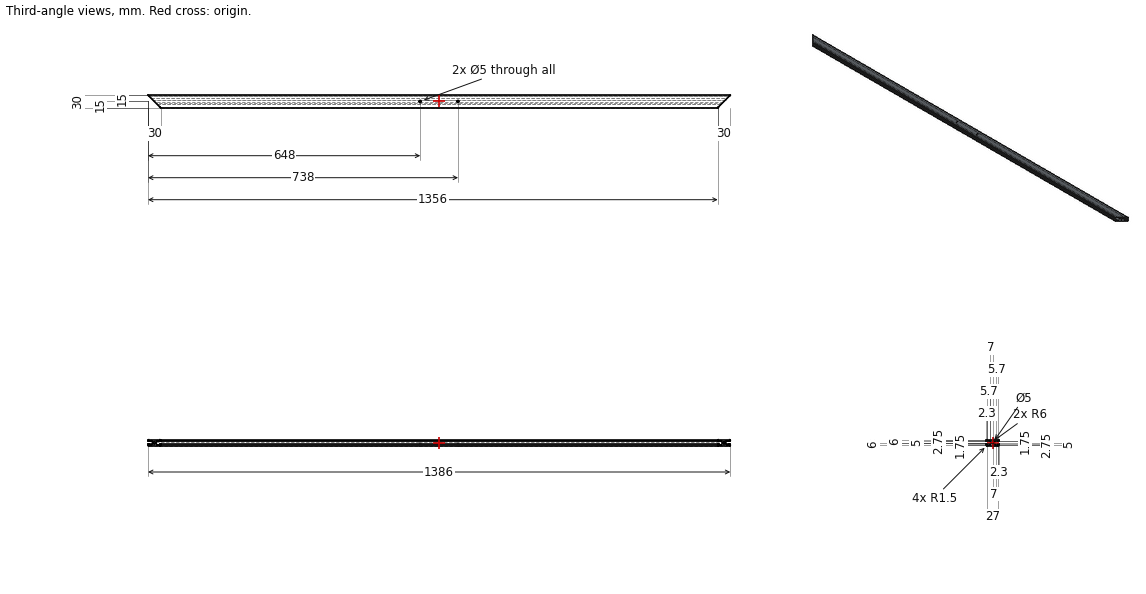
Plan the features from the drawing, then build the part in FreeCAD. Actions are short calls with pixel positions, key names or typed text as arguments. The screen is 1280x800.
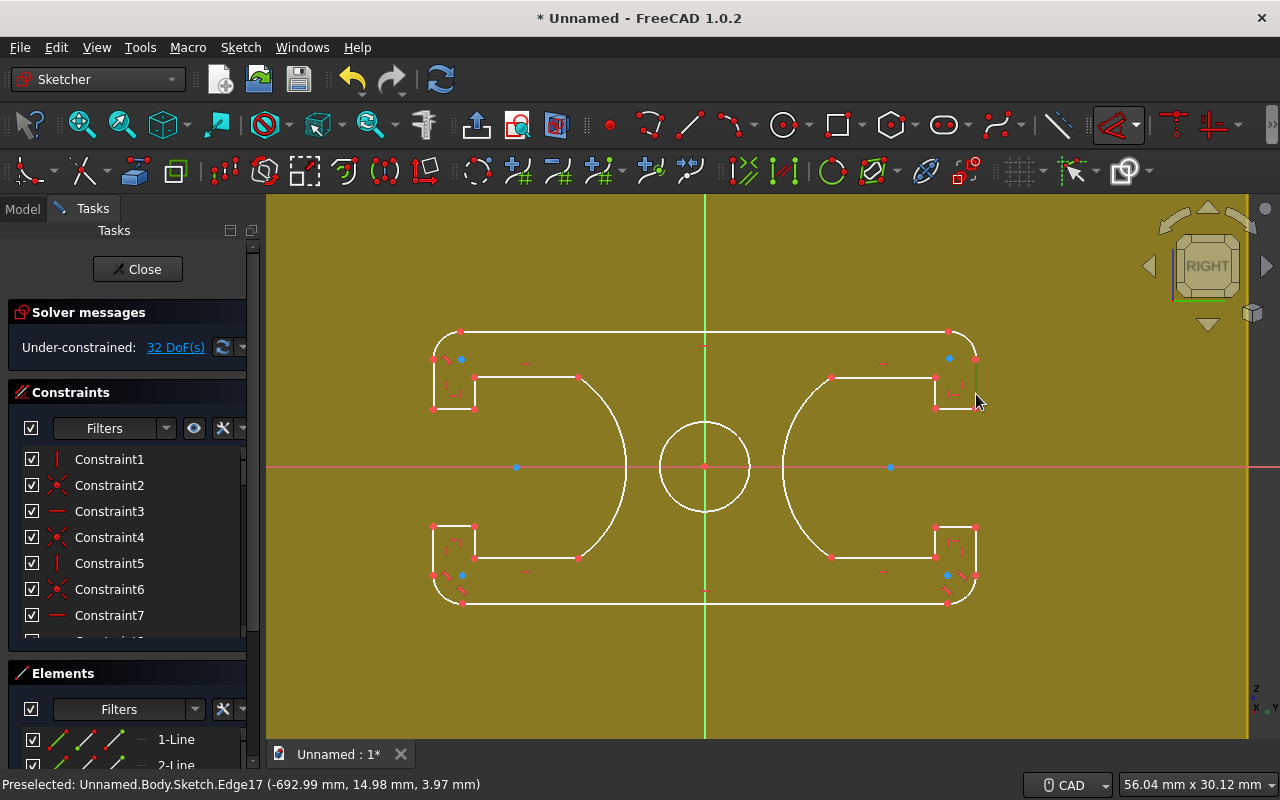
click(973, 347)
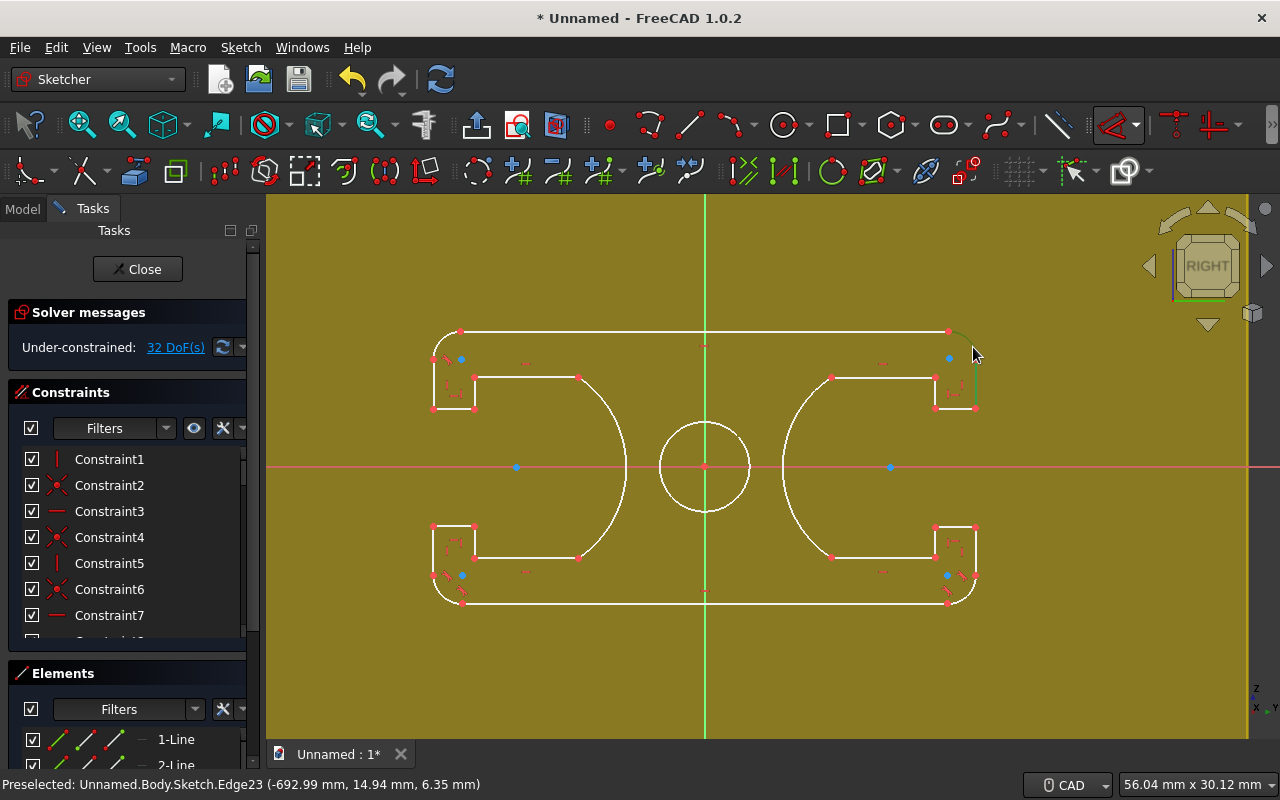
key(t)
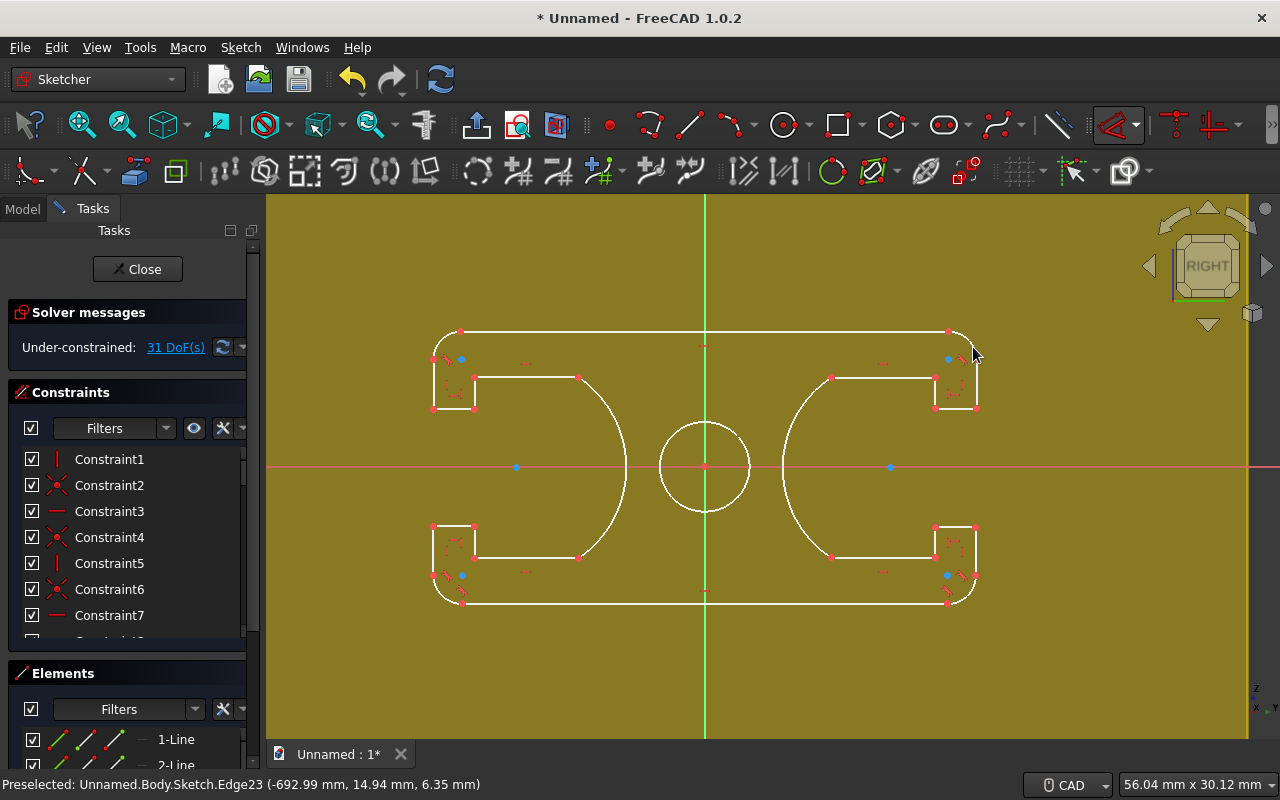
click(803, 332)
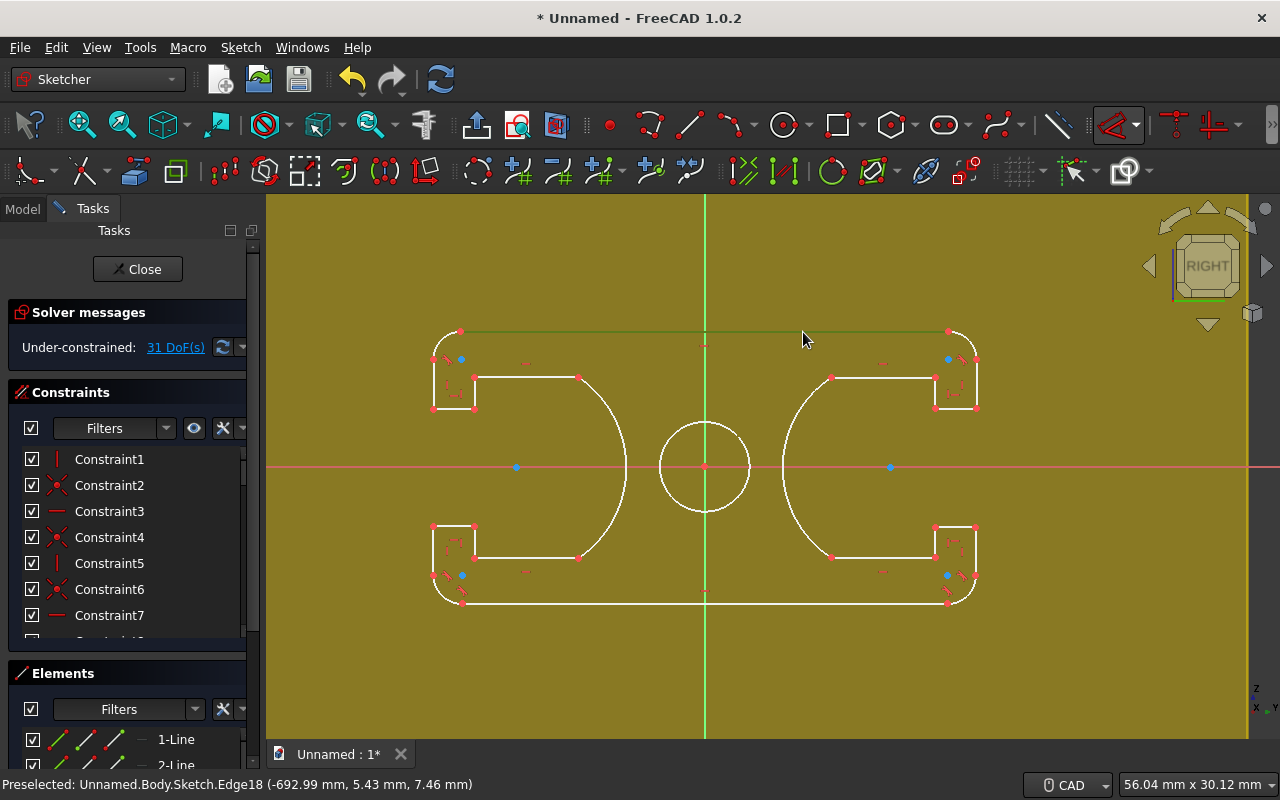
click(974, 347)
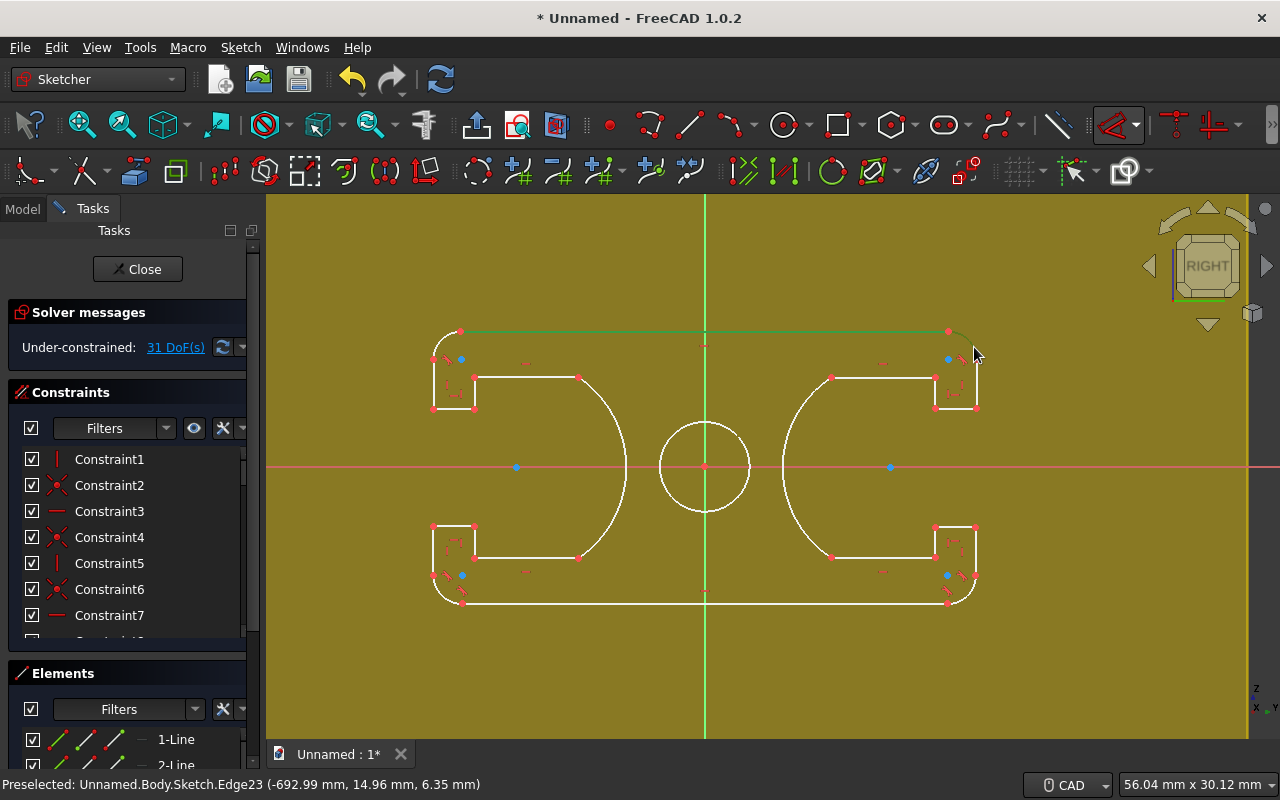
key(t)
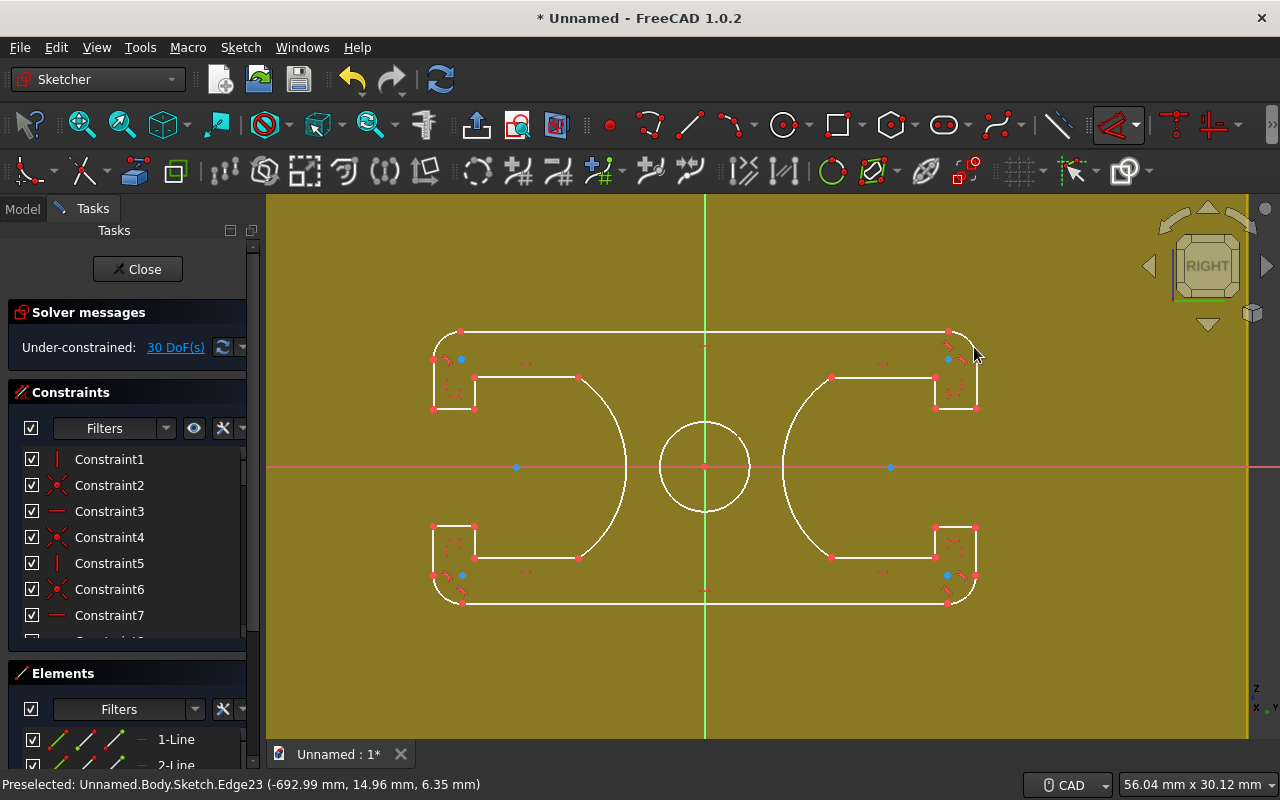
click(802, 332)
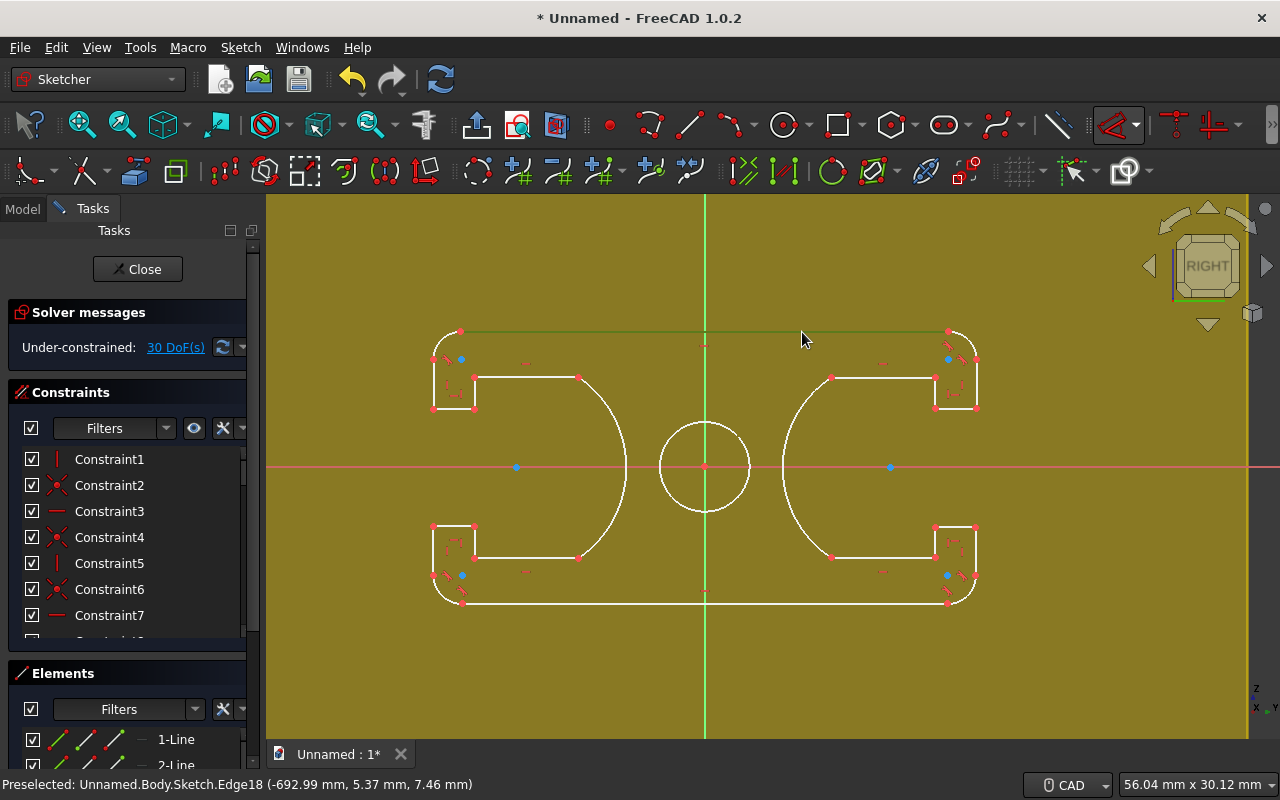
click(448, 335)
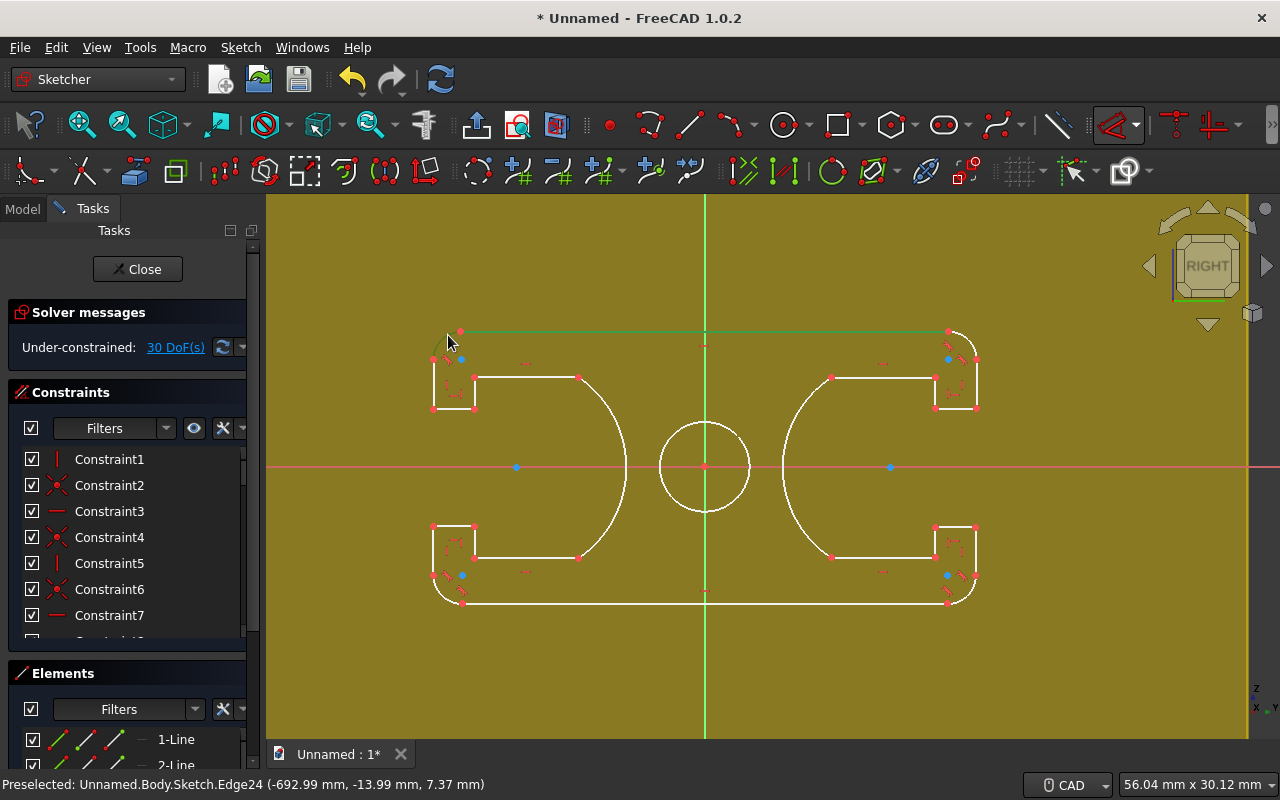
key(t)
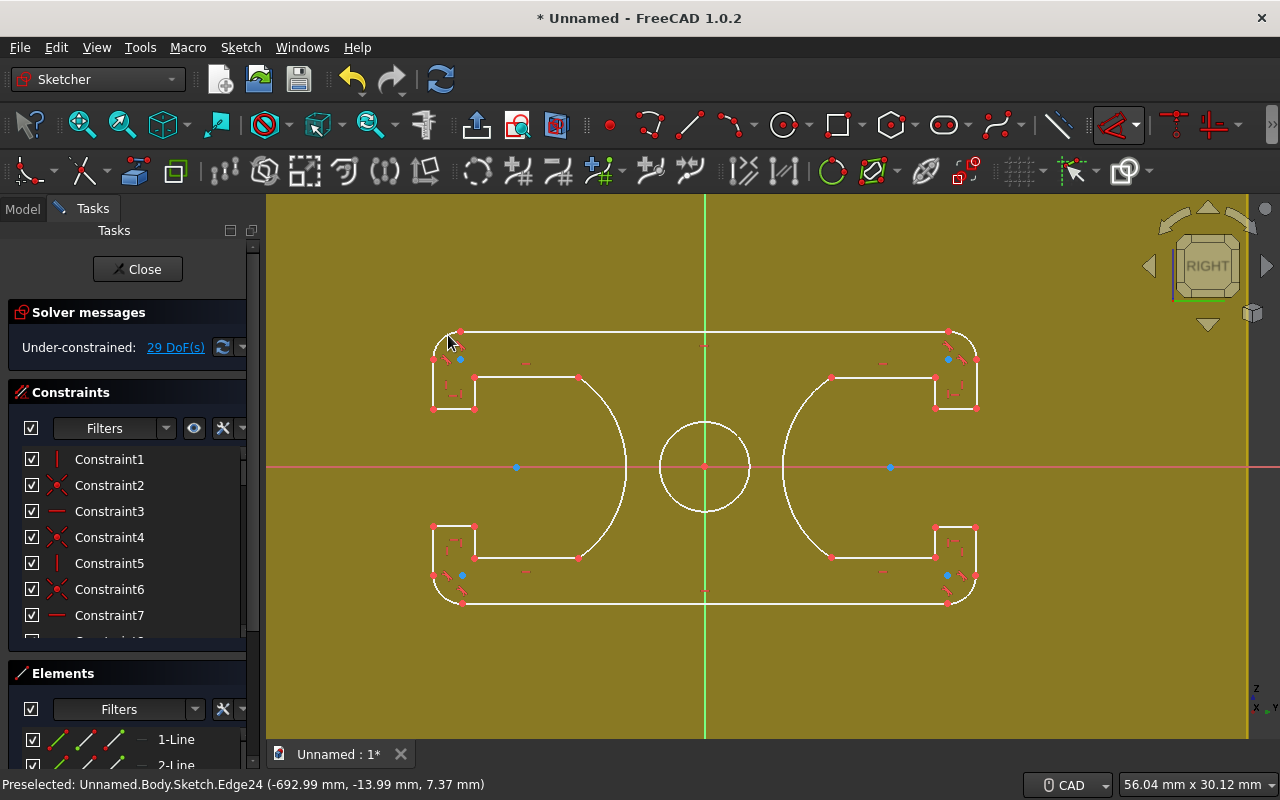
click(437, 588)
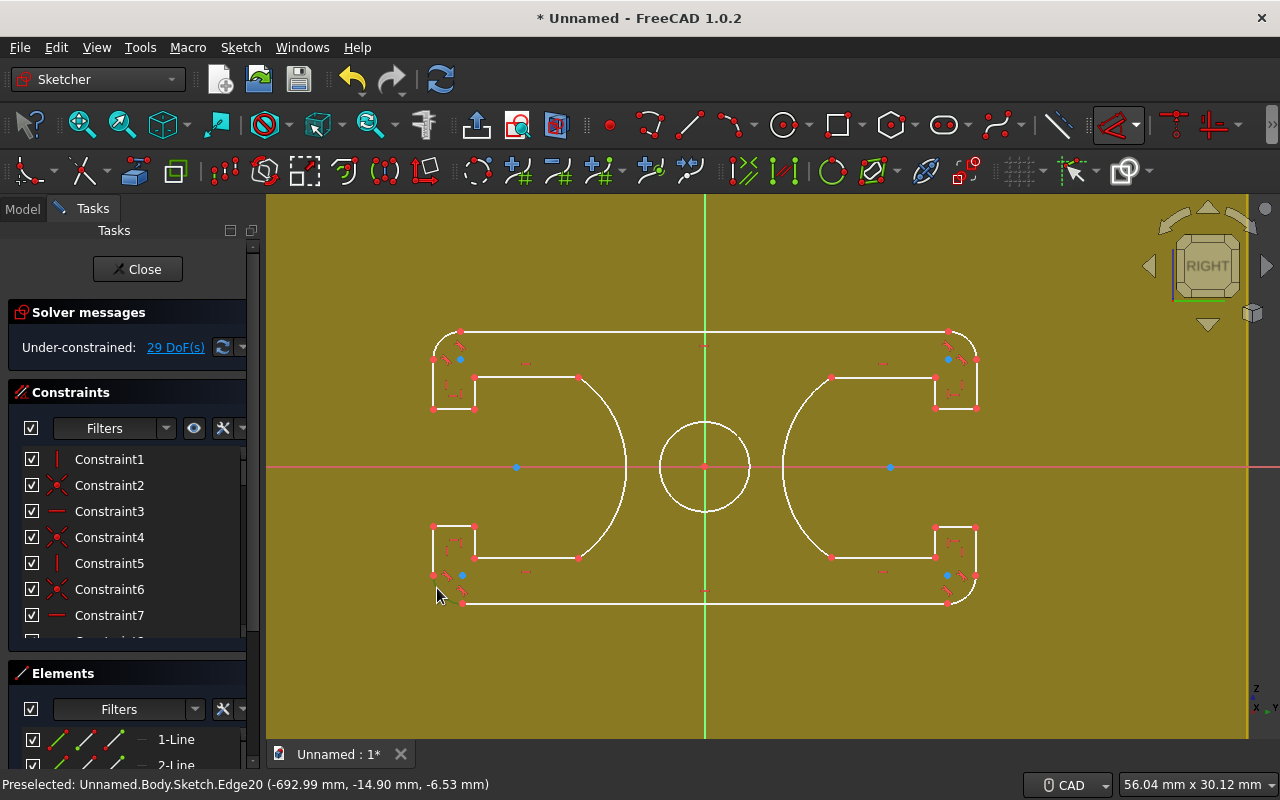
click(961, 601)